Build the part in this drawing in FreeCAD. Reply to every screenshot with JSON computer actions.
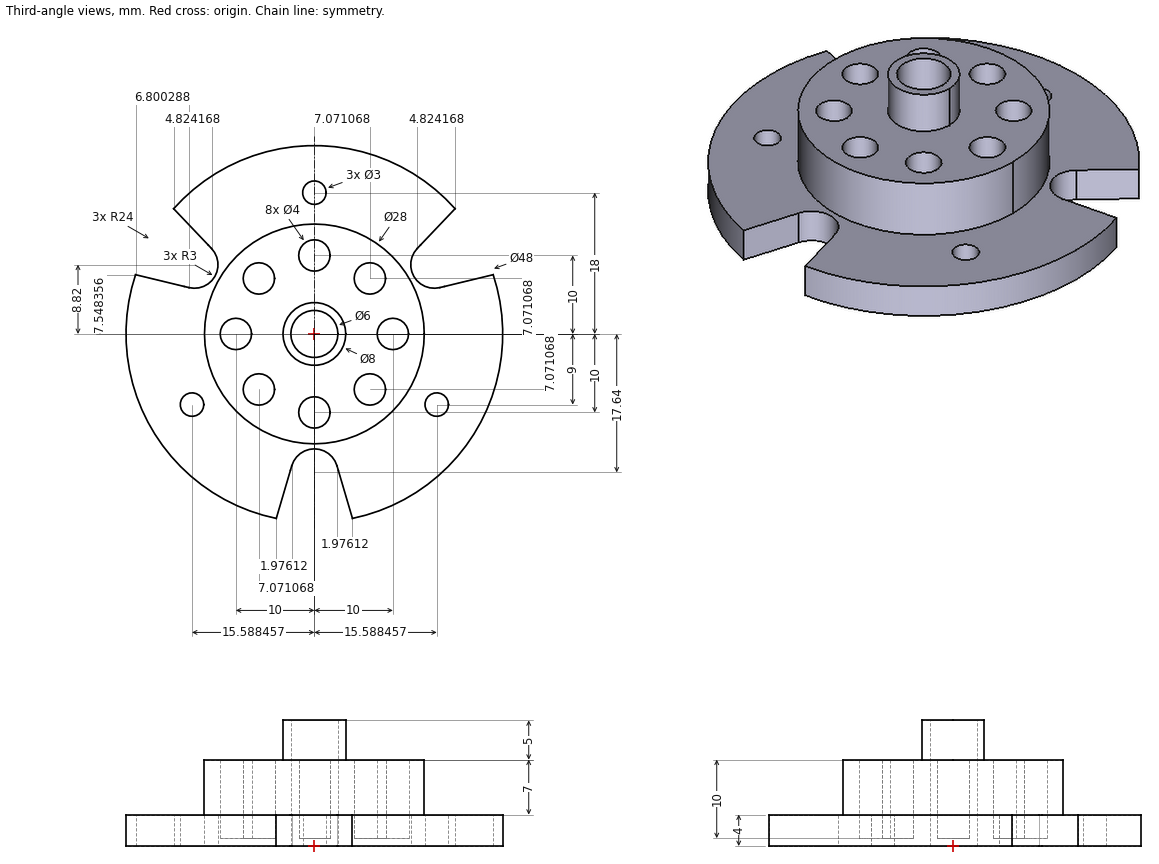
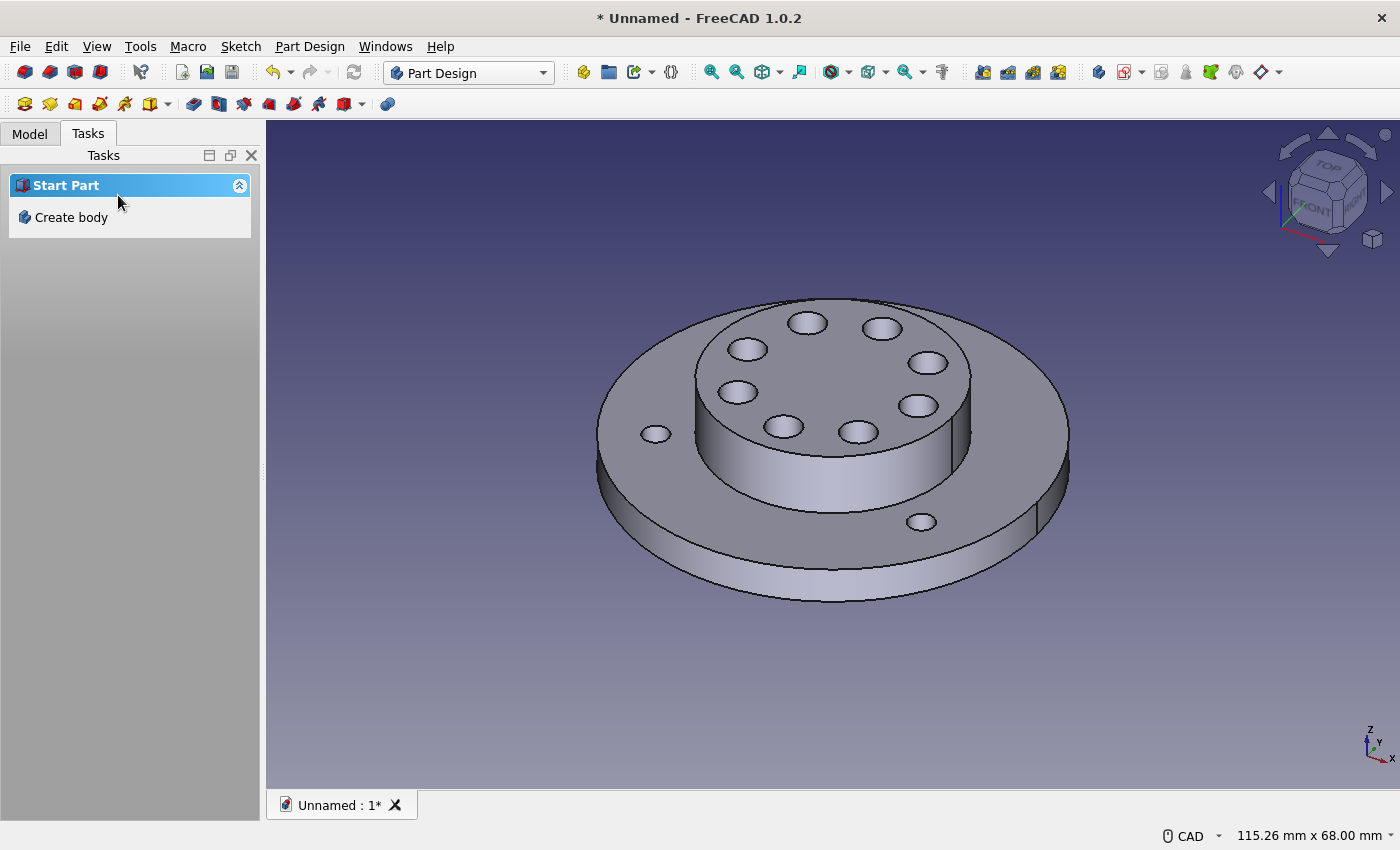
{"action": "left_click", "coordinate": [833, 377]}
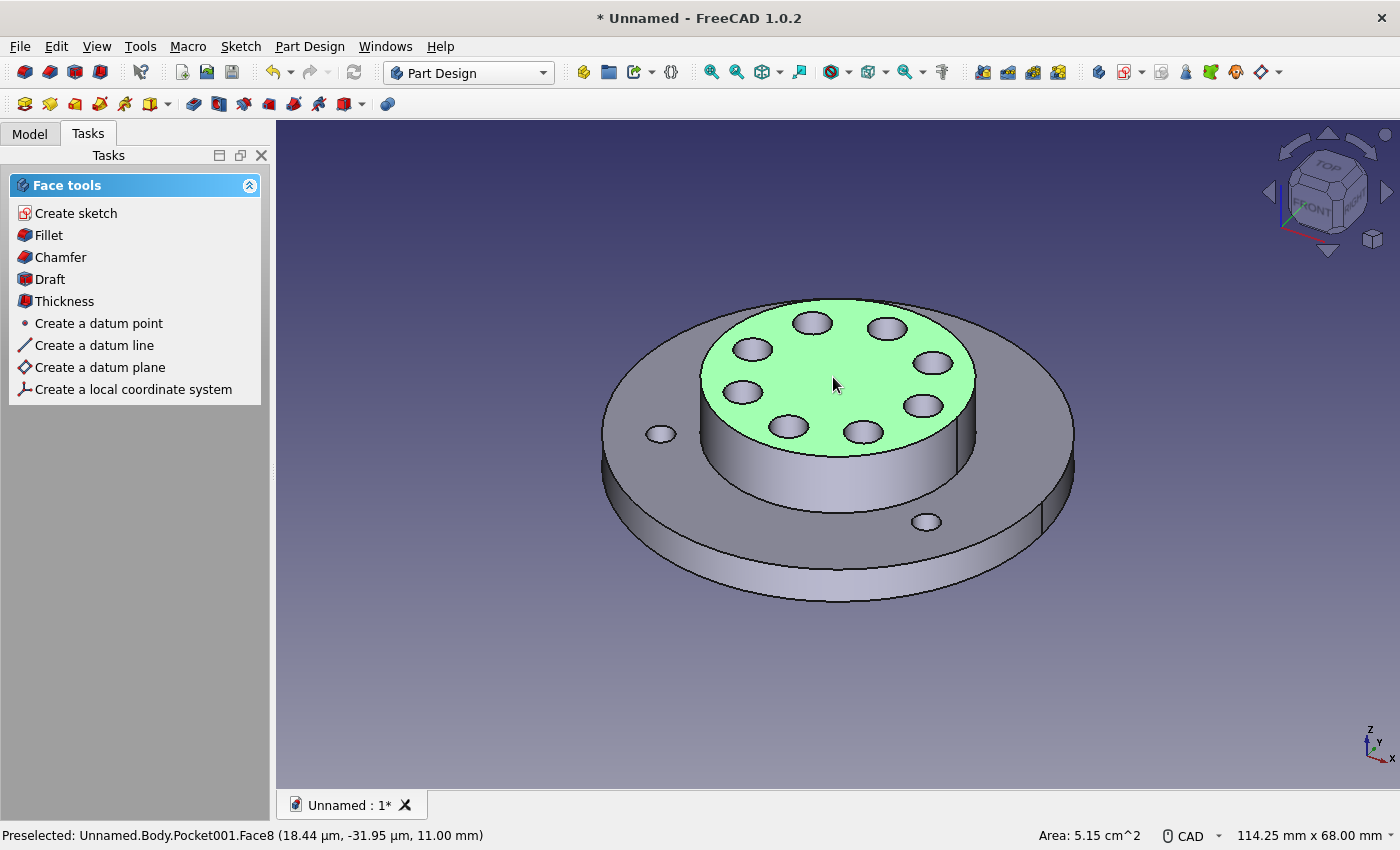
{"action": "left_click", "coordinate": [1124, 72]}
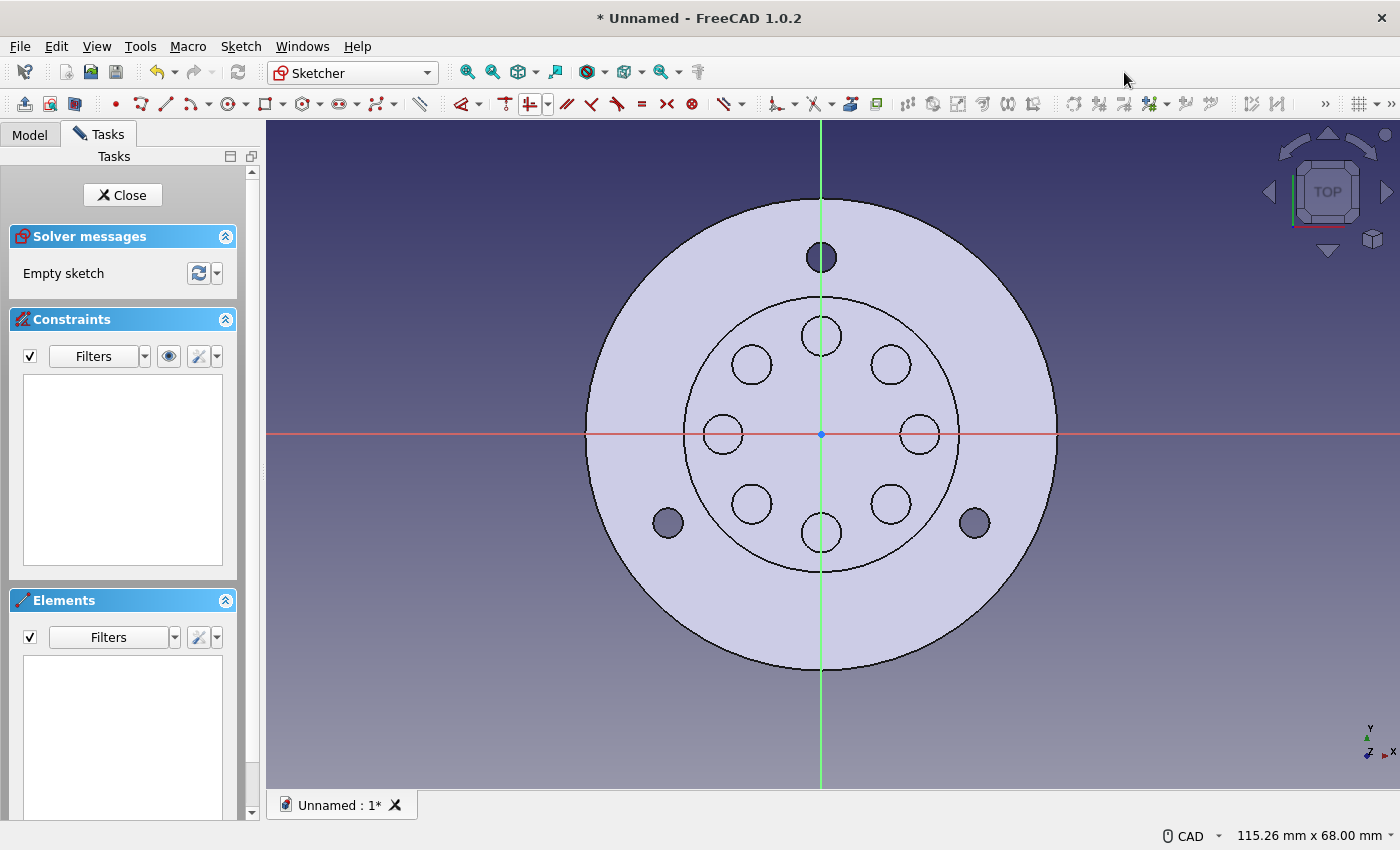
{"action": "scroll", "coordinate": [833, 431], "scroll_direction": "up", "scroll_amount": 9}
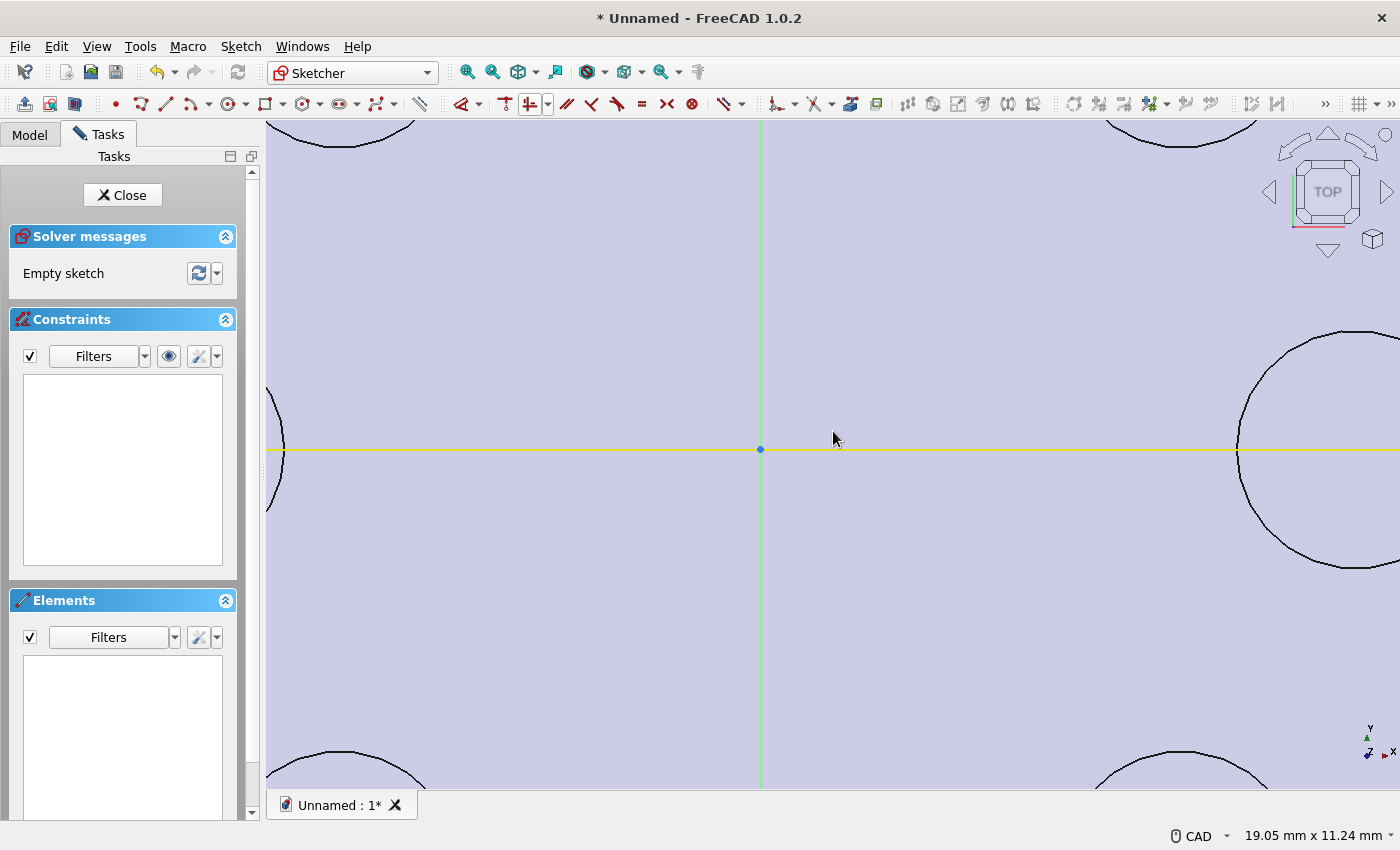
{"action": "left_click", "coordinate": [228, 104]}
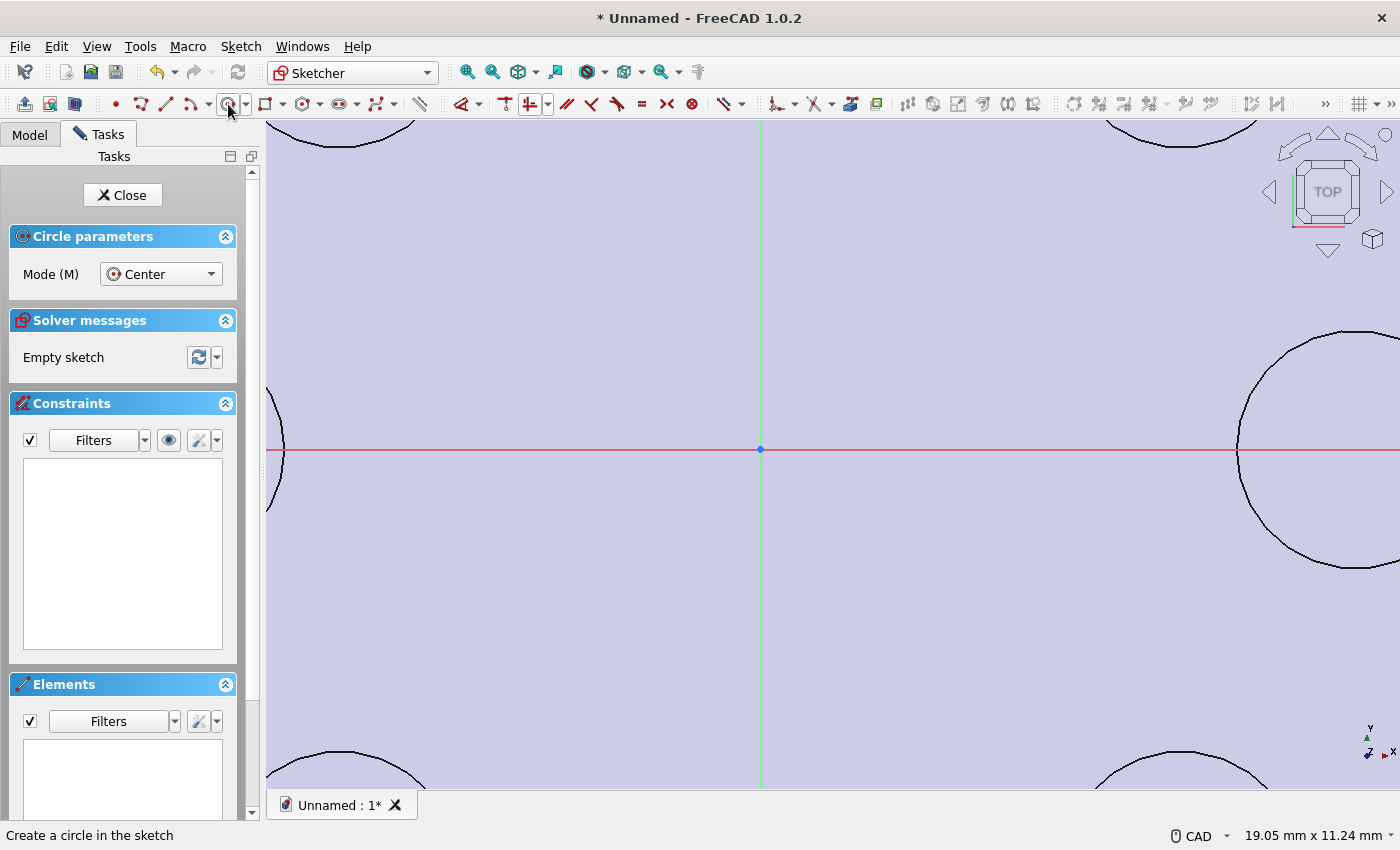
{"action": "left_click", "coordinate": [761, 450]}
{"action": "mouse_move", "coordinate": [929, 281]}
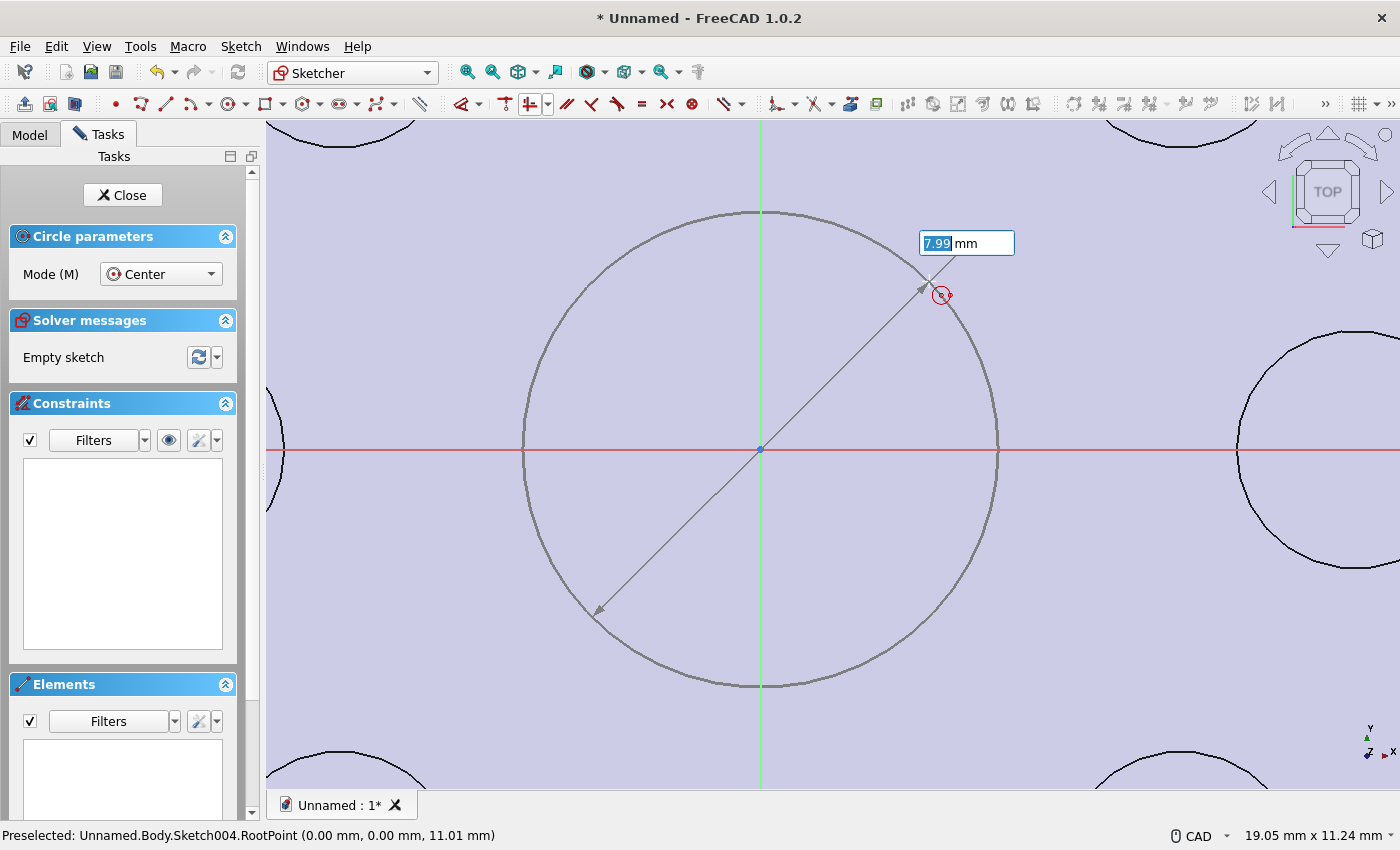
{"action": "type", "text": "8"}
{"action": "key", "text": "Return"}
{"action": "key", "text": "Escape"}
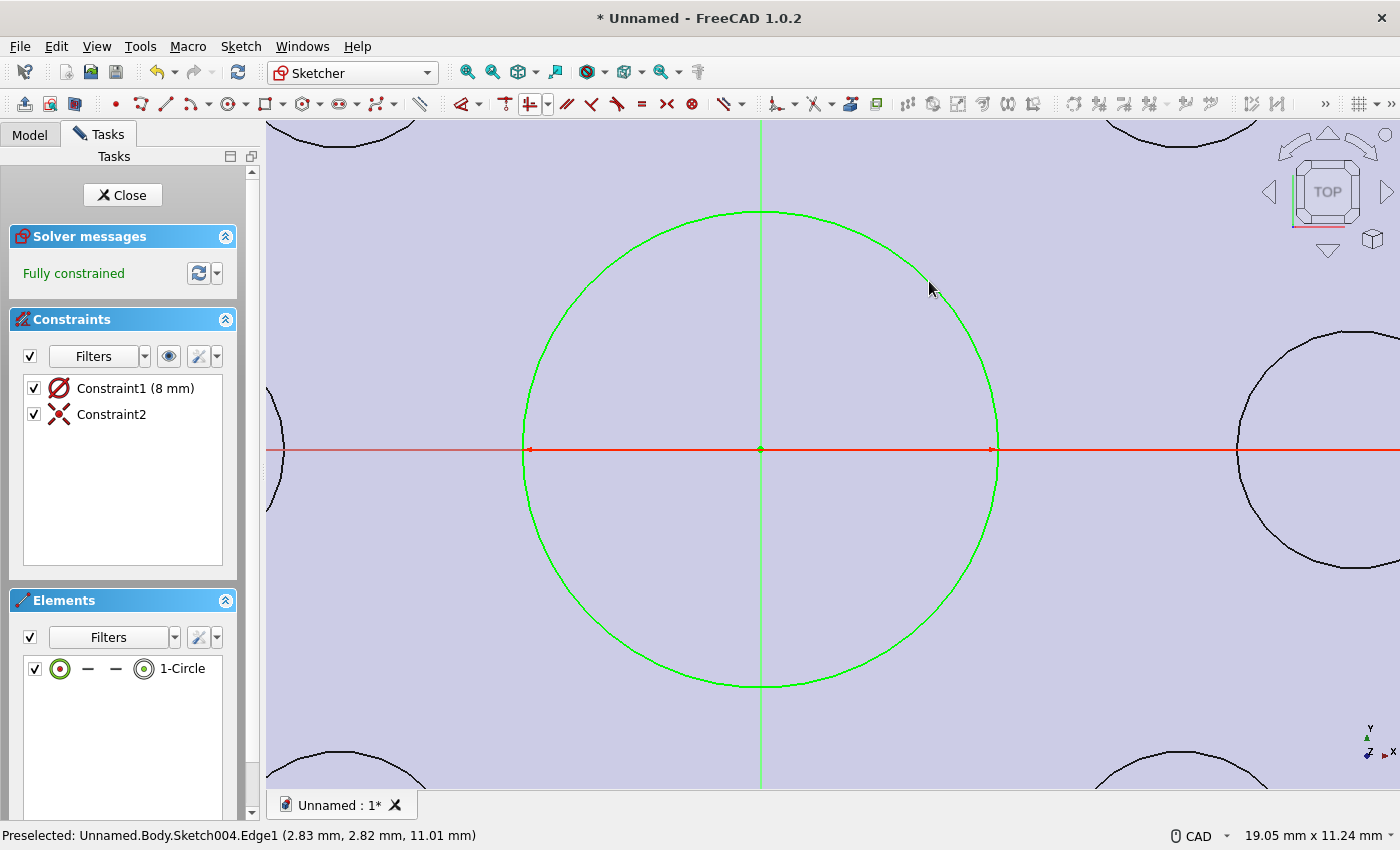
{"action": "left_click", "coordinate": [123, 195]}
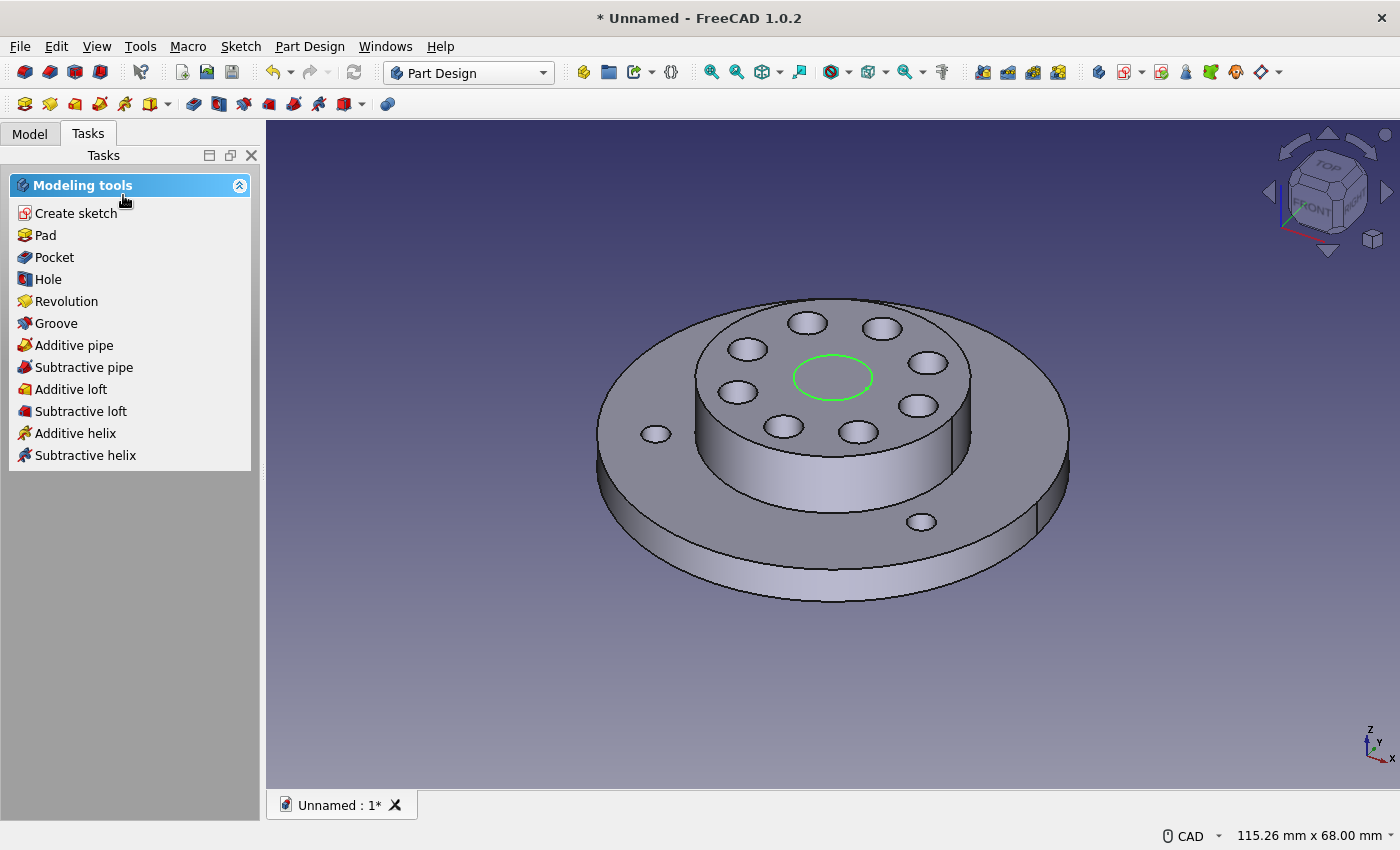
{"action": "left_click", "coordinate": [25, 104]}